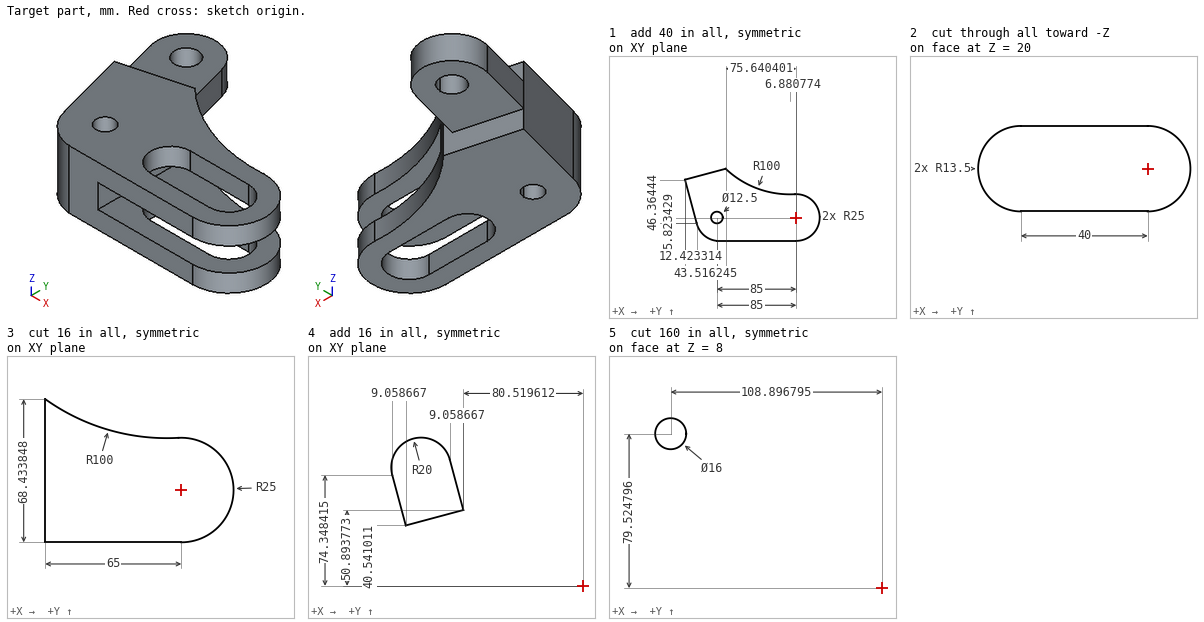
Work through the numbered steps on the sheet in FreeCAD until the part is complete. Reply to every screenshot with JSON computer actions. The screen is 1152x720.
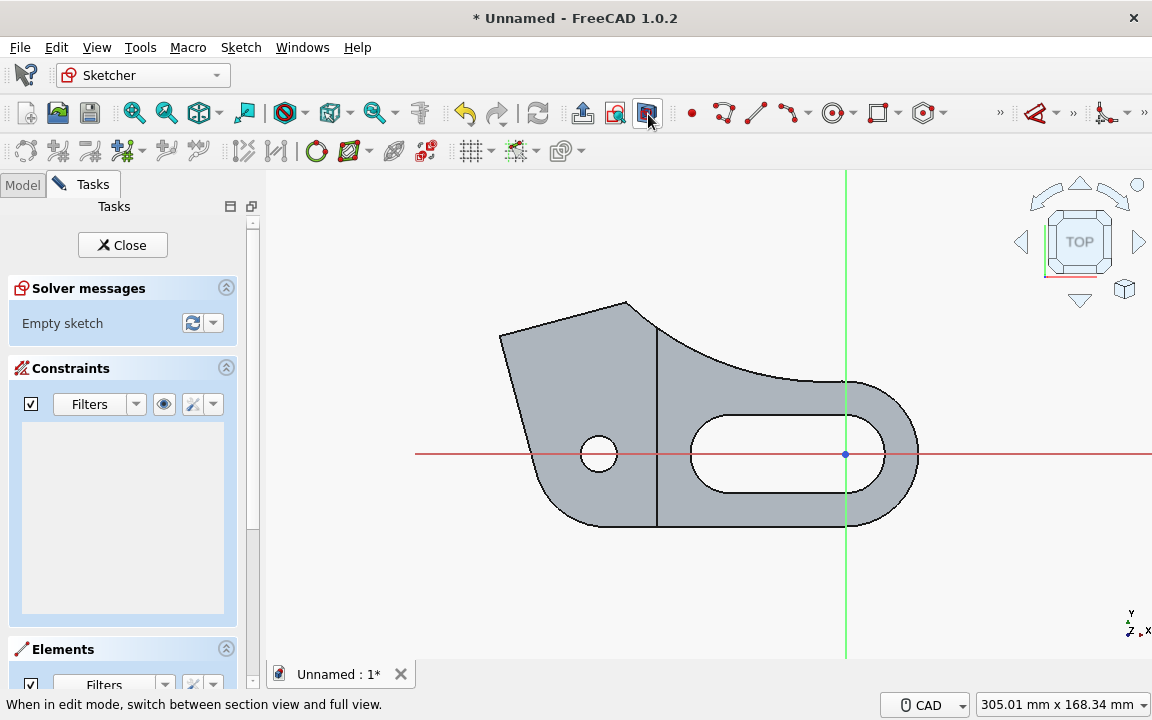
{"action": "scroll", "coordinate": [554, 631], "scroll_direction": "down", "scroll_amount": 1}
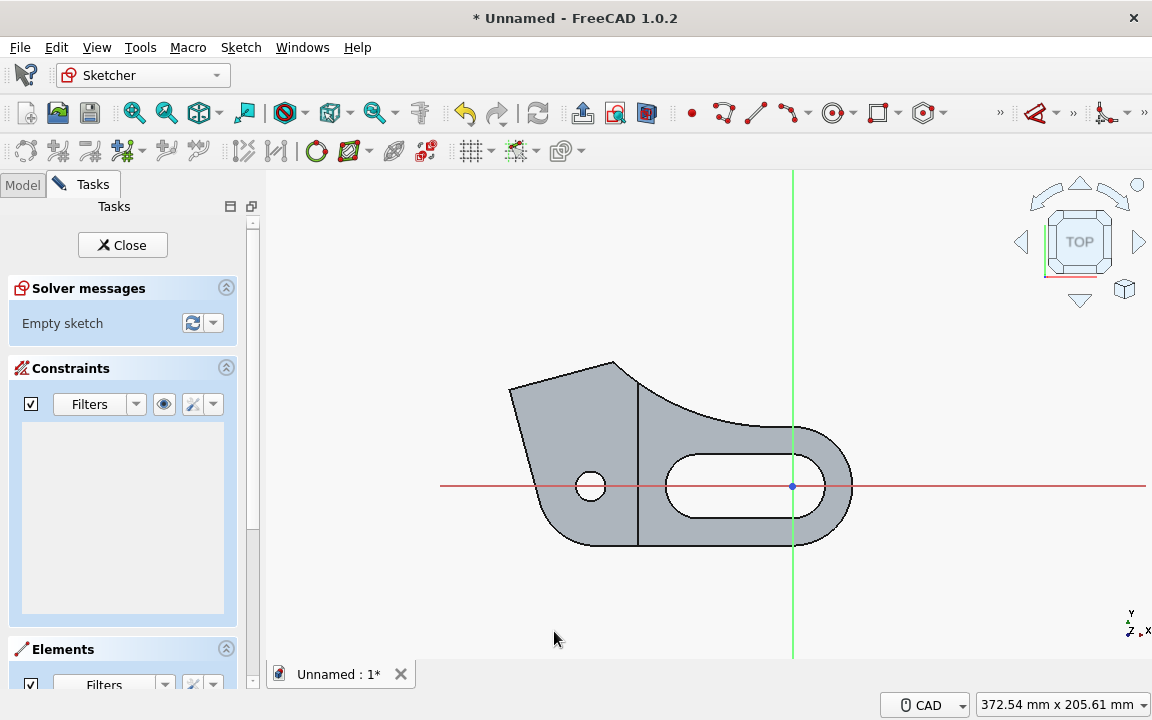
{"action": "left_click", "coordinate": [724, 114]}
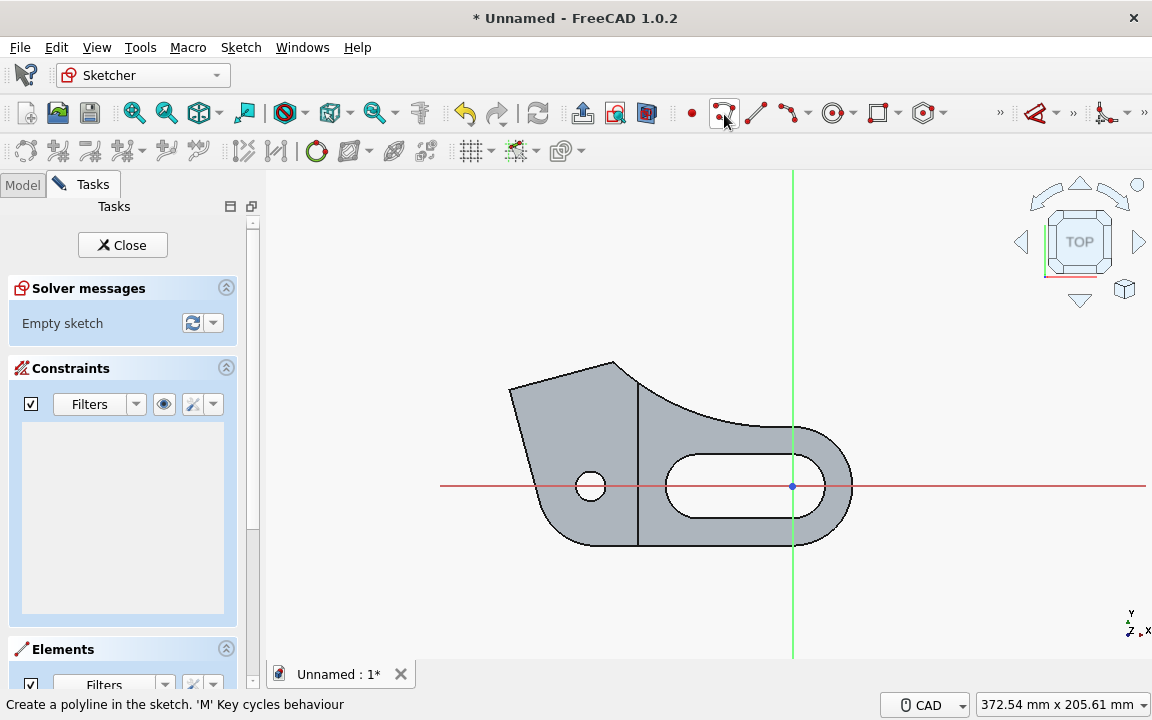
{"action": "left_click", "coordinate": [488, 309]}
{"action": "left_click", "coordinate": [510, 390]}
{"action": "left_click", "coordinate": [601, 365]}
{"action": "left_click", "coordinate": [580, 285]}
{"action": "right_click", "coordinate": [580, 285]}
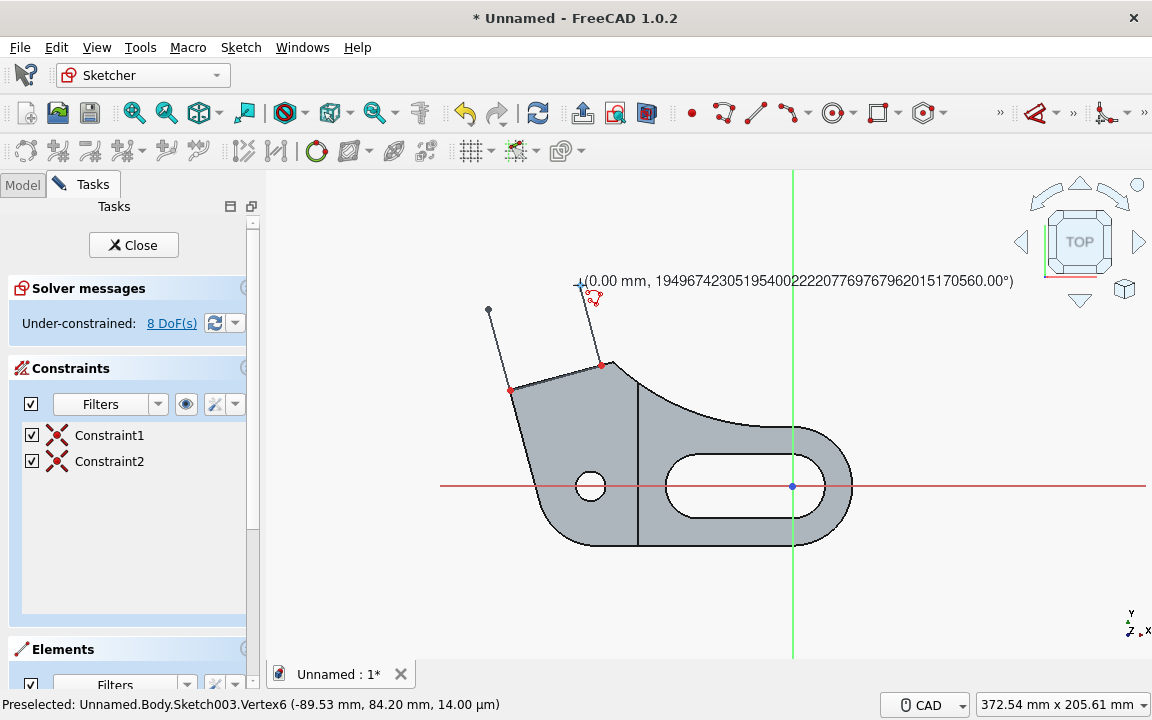
{"action": "left_click", "coordinate": [788, 114]}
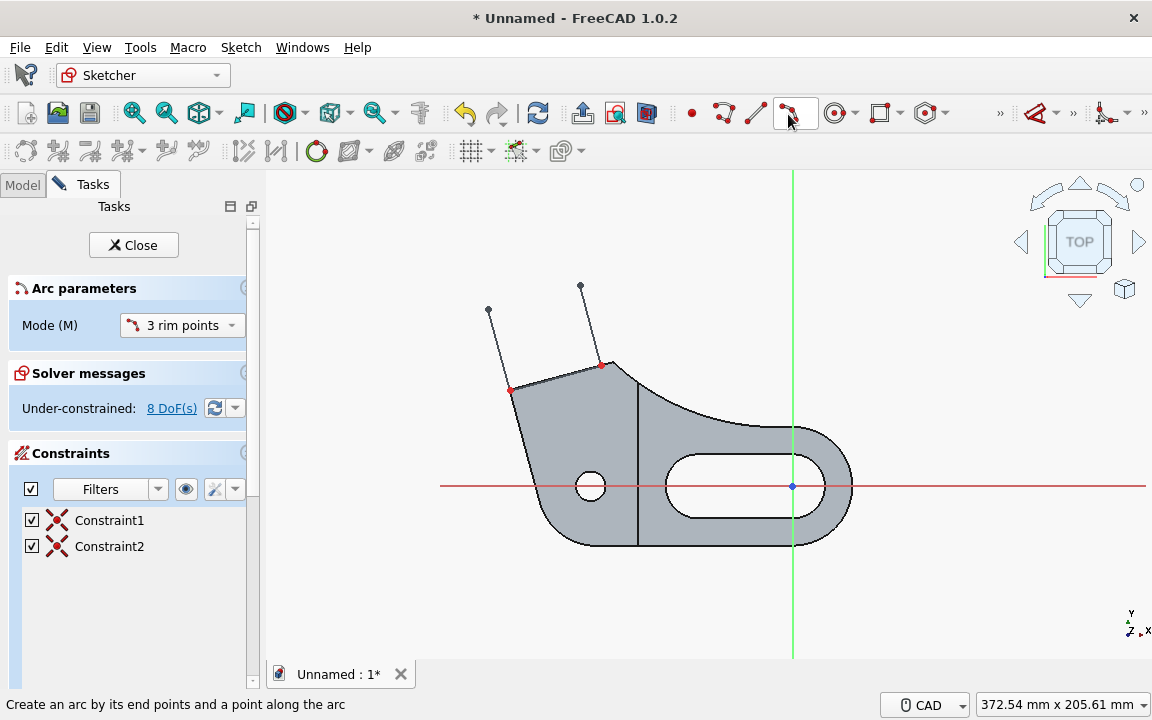
{"action": "left_click", "coordinate": [580, 286]}
{"action": "left_click", "coordinate": [488, 310]}
{"action": "left_click", "coordinate": [522, 251]}
{"action": "key", "text": "Escape"}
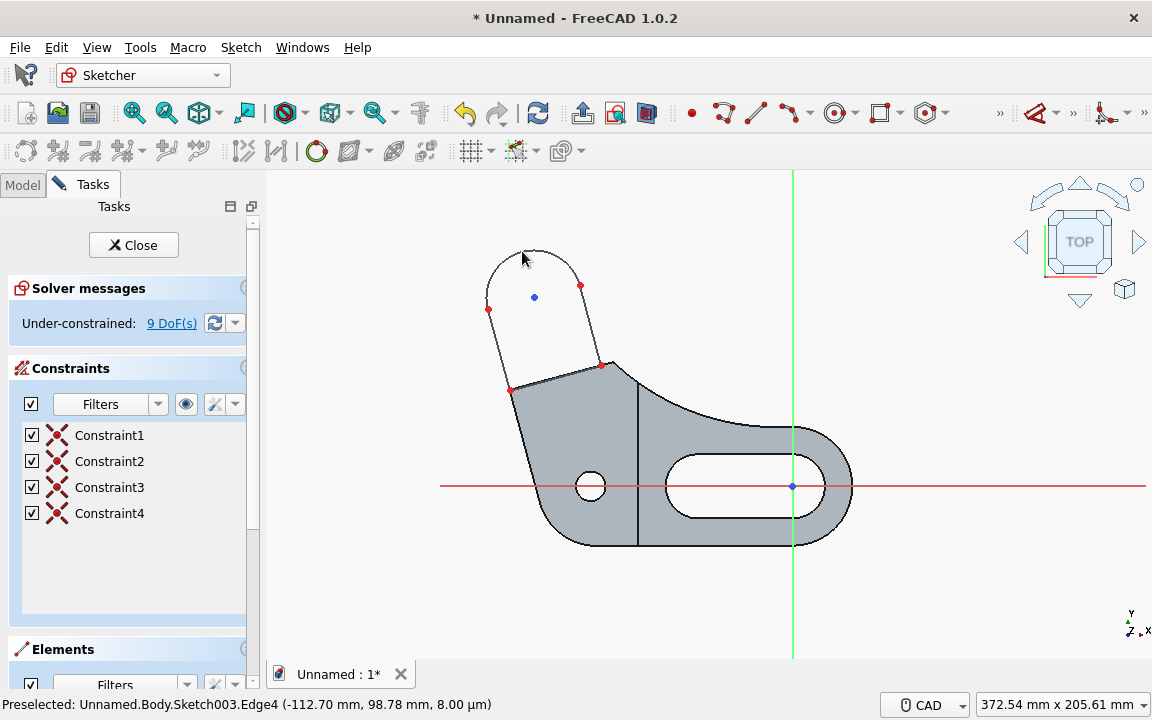
{"action": "left_click", "coordinate": [495, 334]}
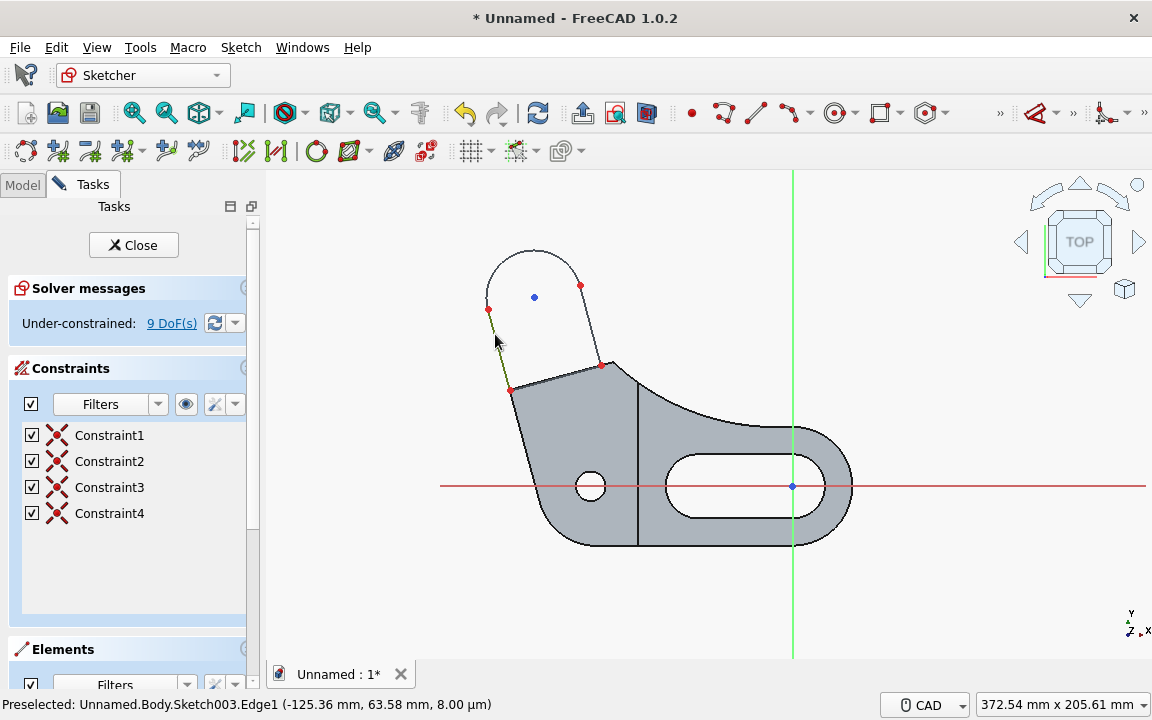
{"action": "left_click", "coordinate": [551, 254]}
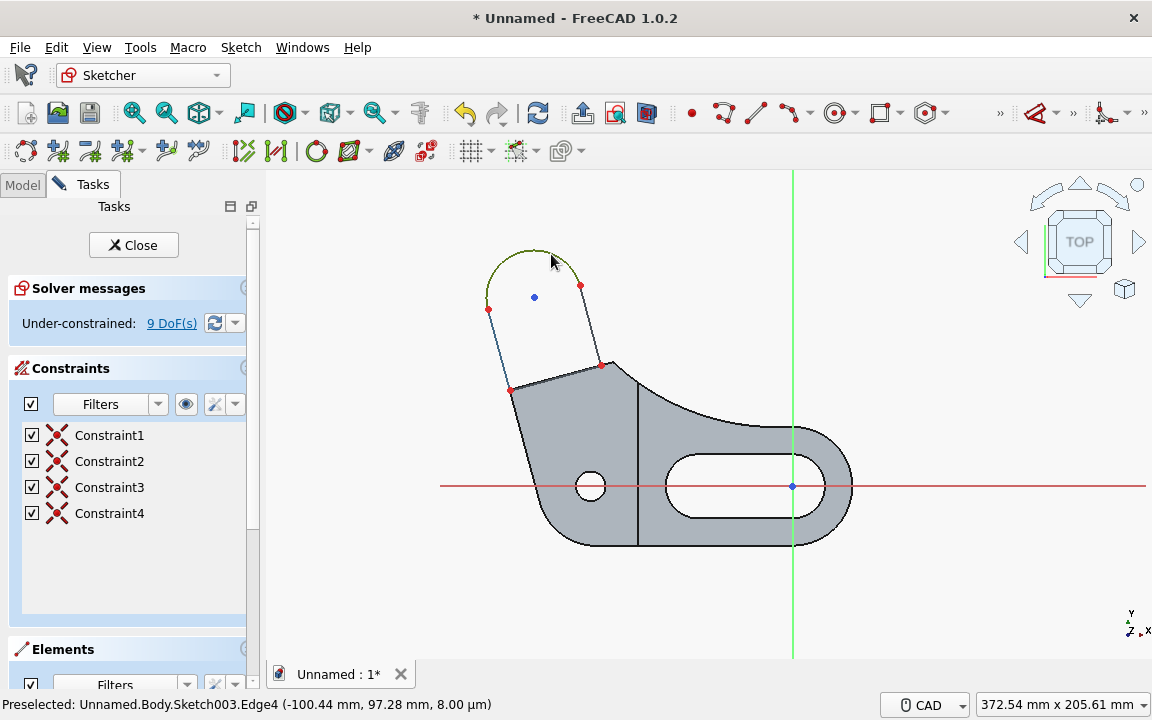
{"action": "key", "text": "t"}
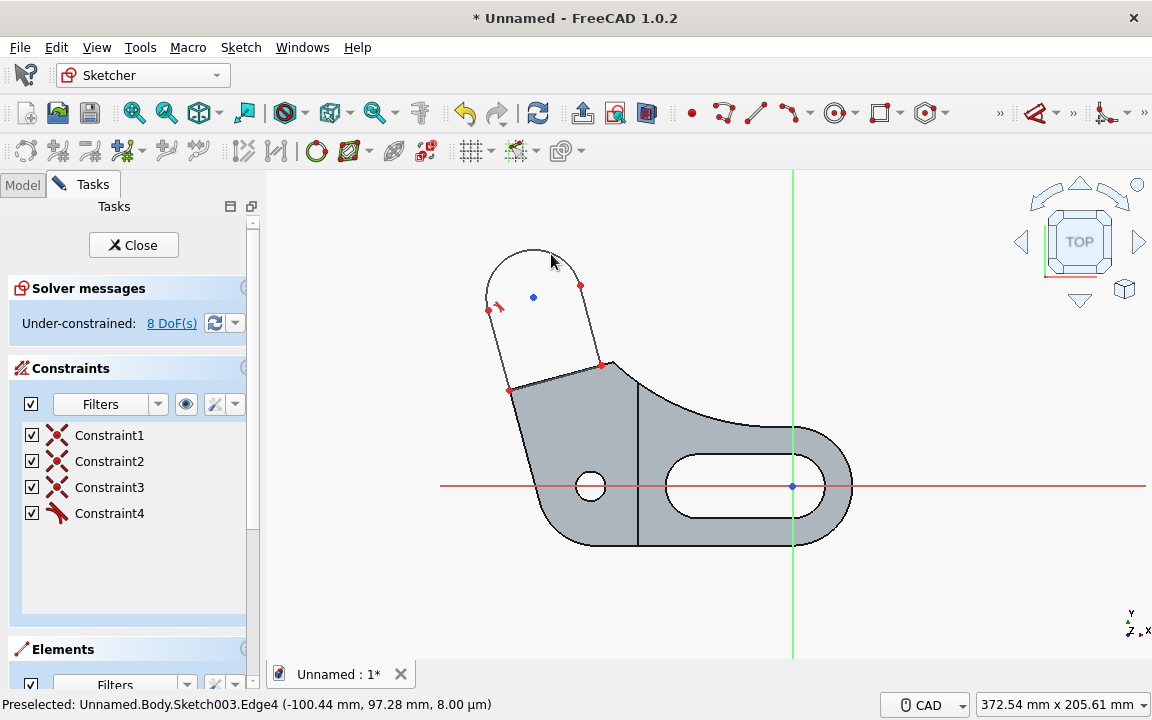
{"action": "left_click", "coordinate": [595, 342]}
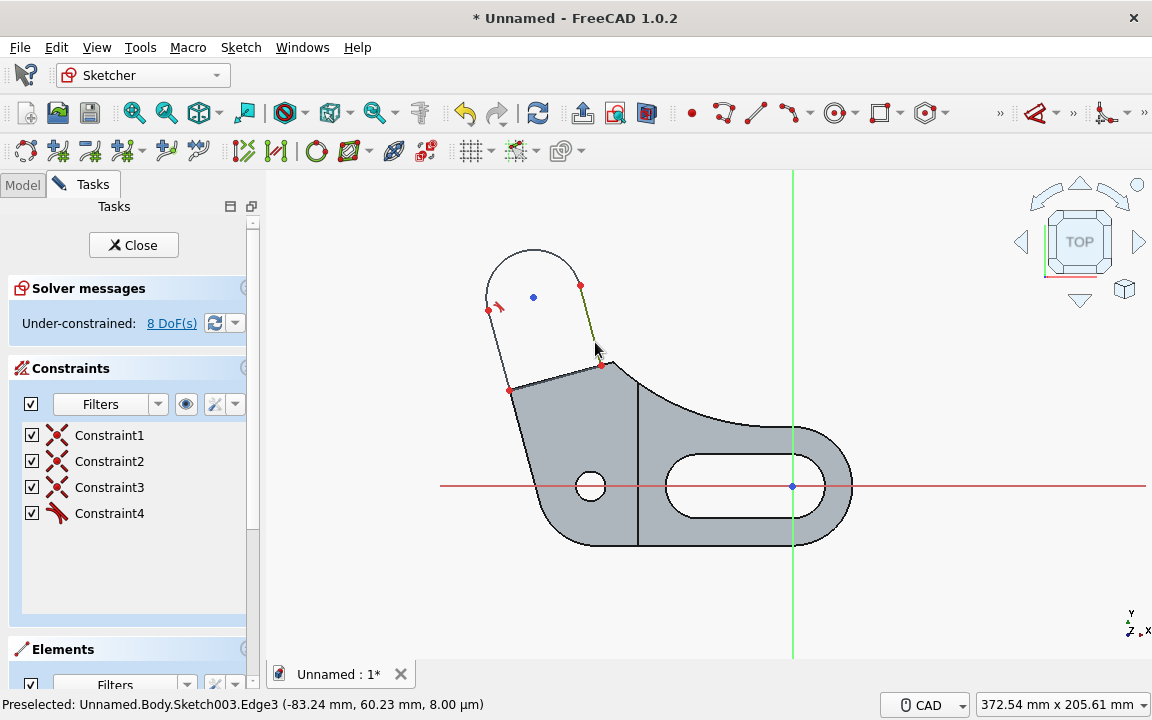
{"action": "left_click", "coordinate": [551, 253]}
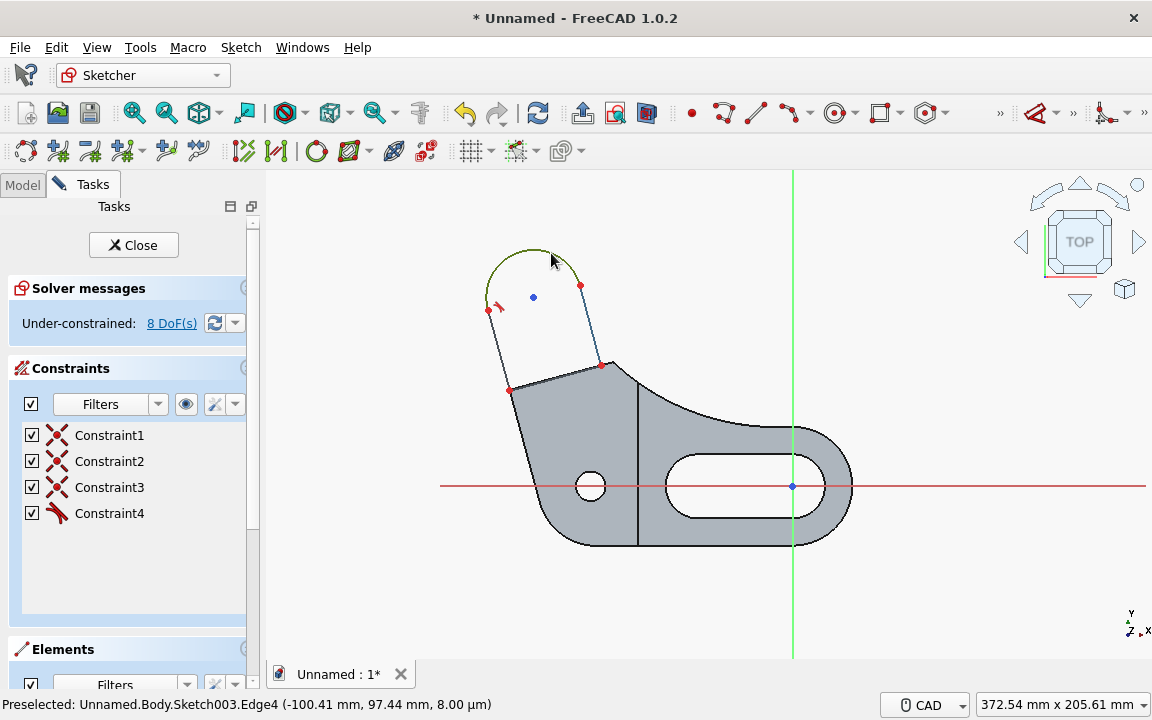
{"action": "key", "text": "t"}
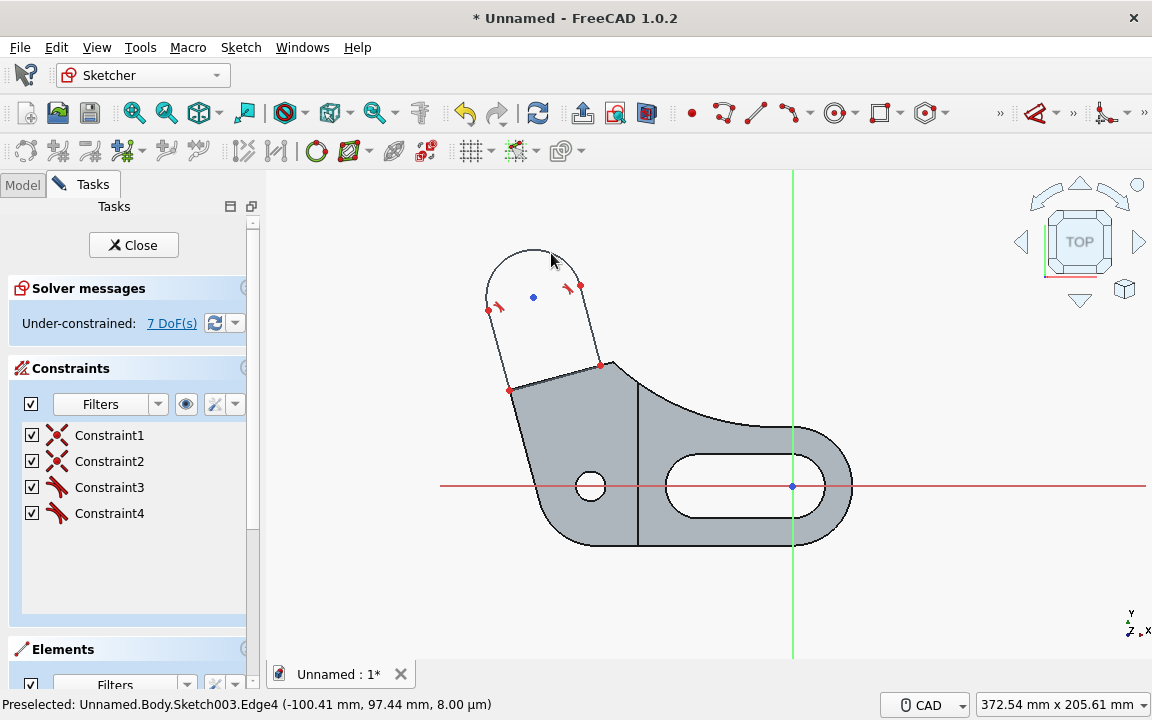
{"action": "left_click", "coordinate": [1036, 114]}